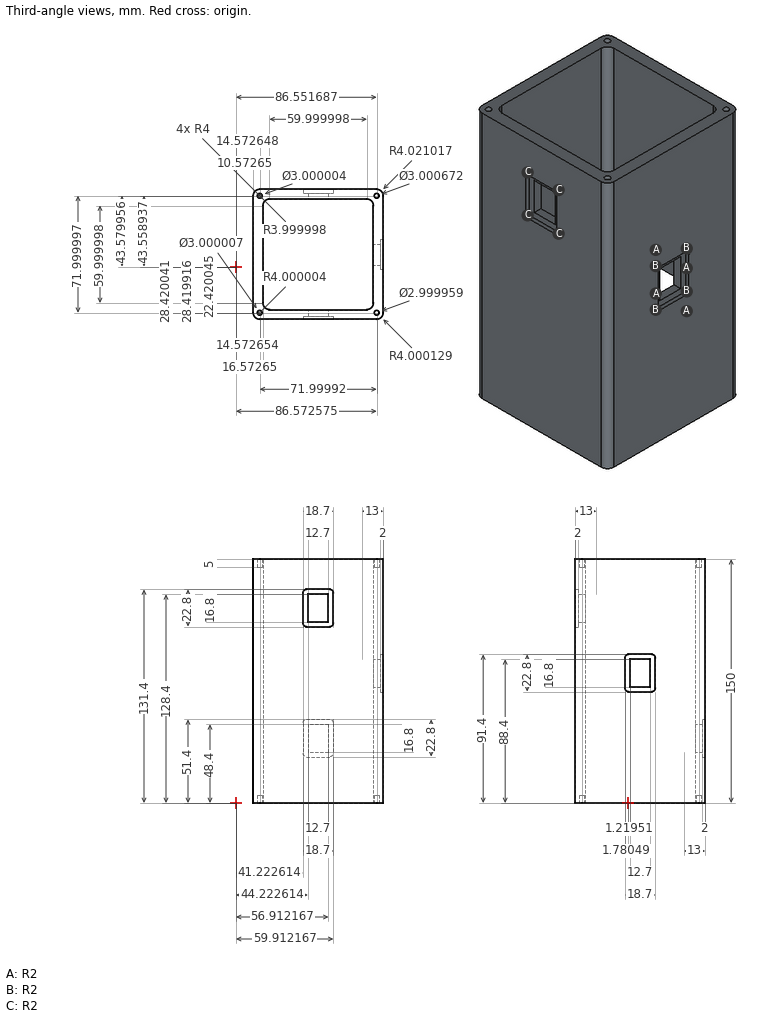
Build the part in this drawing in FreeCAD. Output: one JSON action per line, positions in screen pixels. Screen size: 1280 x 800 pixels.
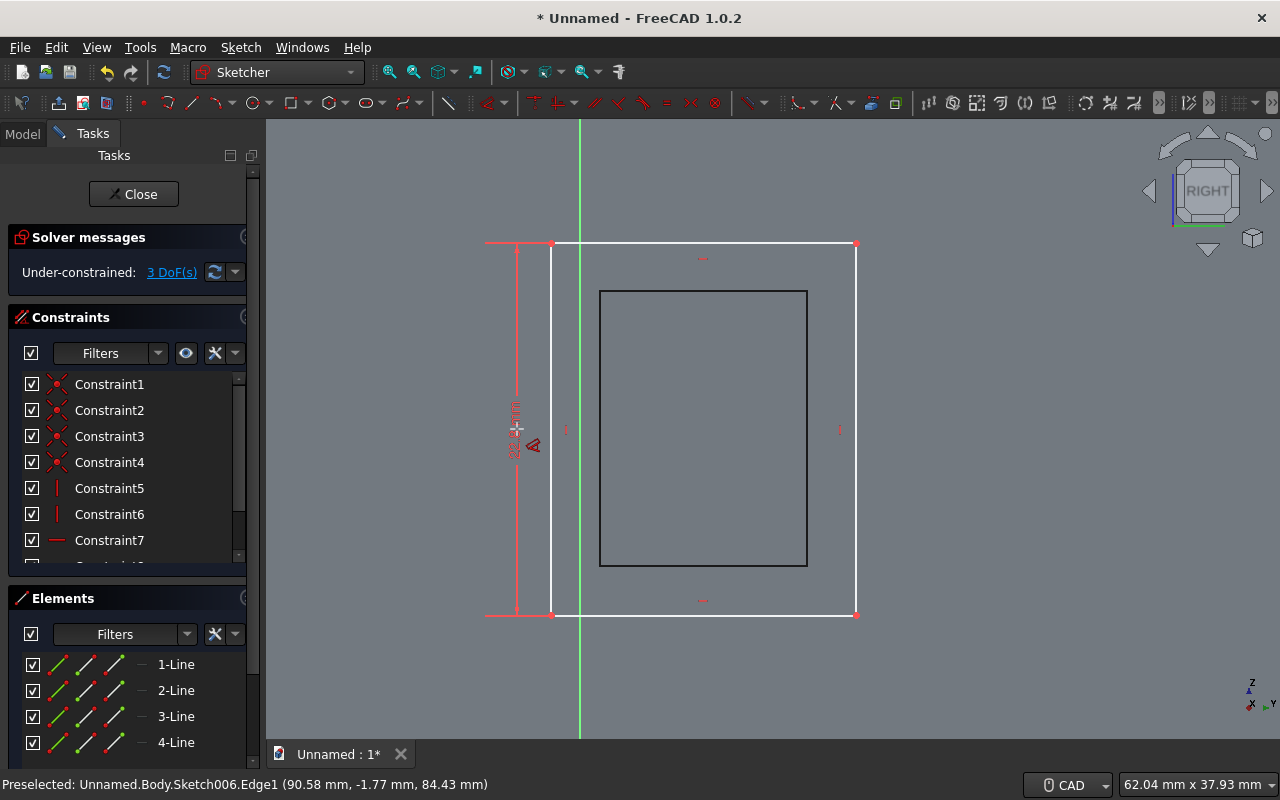
{"action": "left_click", "coordinate": [642, 616]}
{"action": "left_click", "coordinate": [703, 650]}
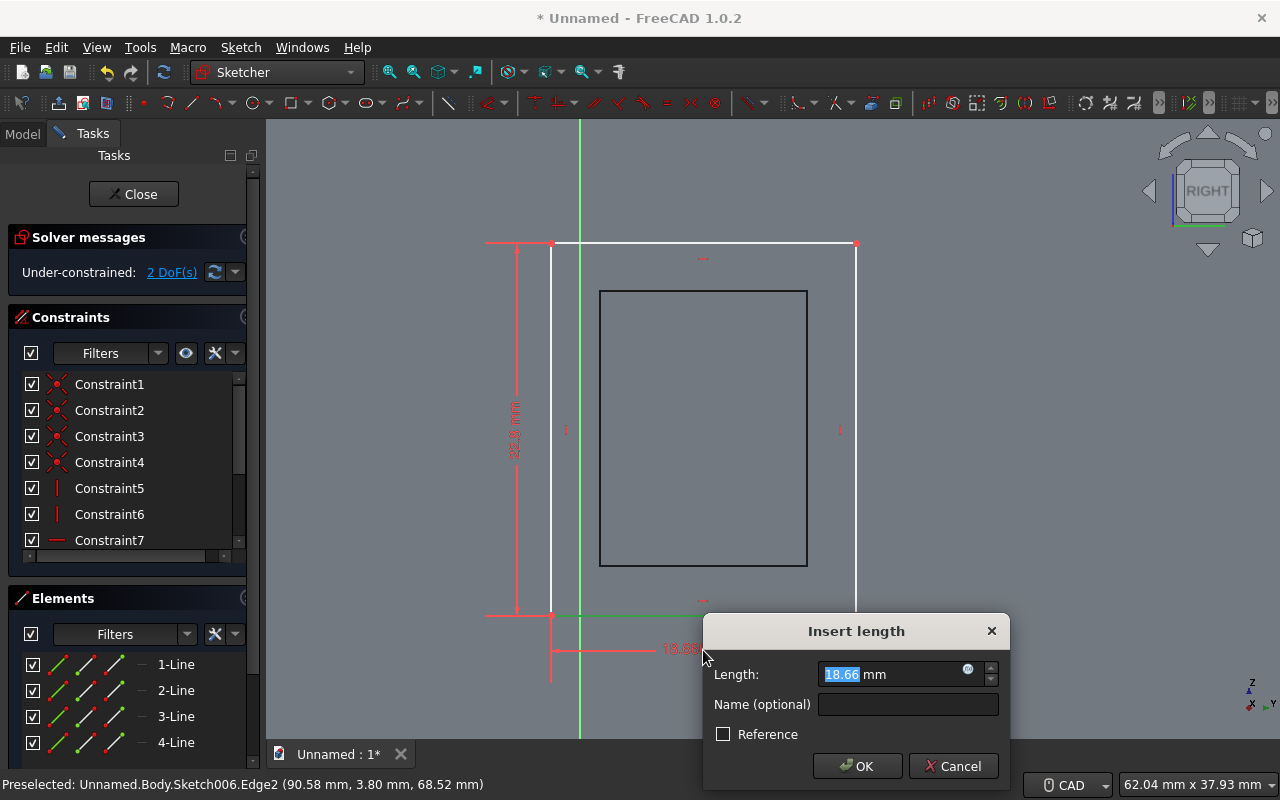
{"action": "type", "text": "18.7"}
{"action": "key", "text": "Return"}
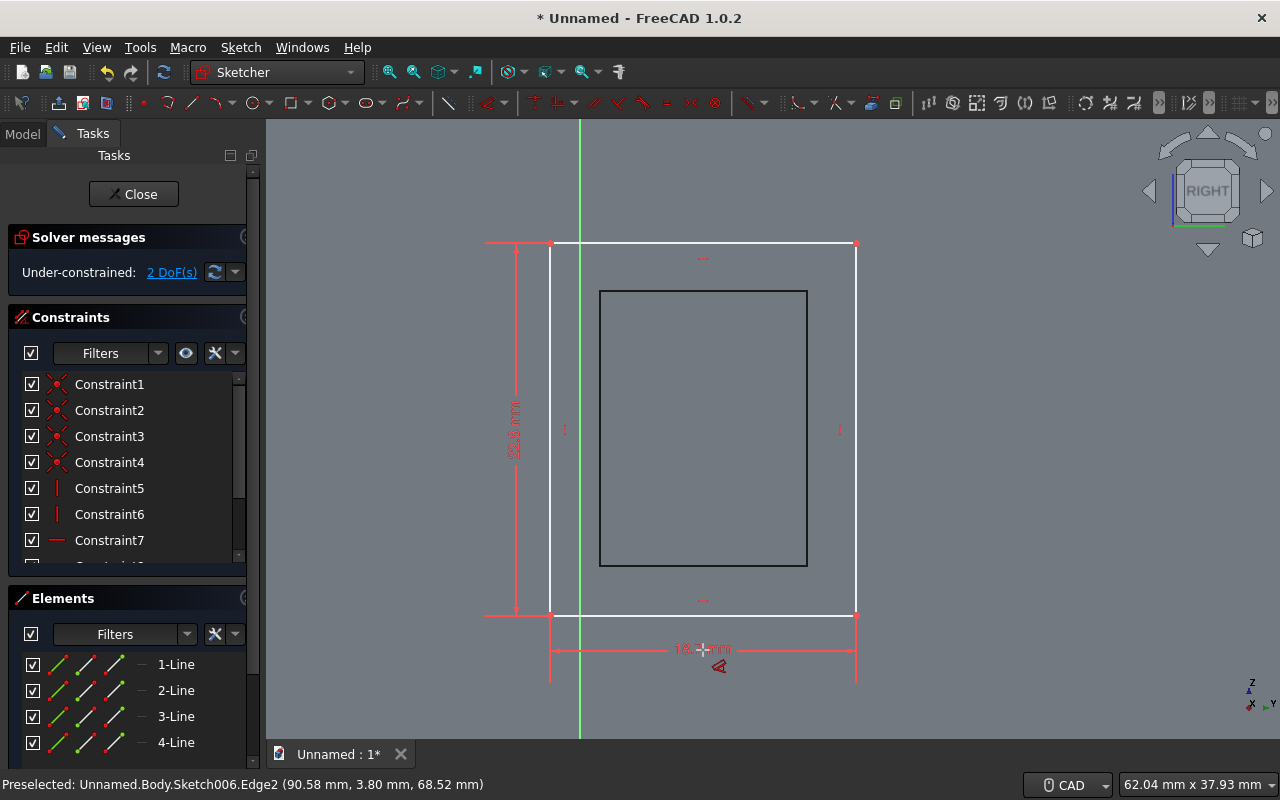
{"action": "left_click", "coordinate": [550, 243]}
{"action": "left_click", "coordinate": [516, 477]}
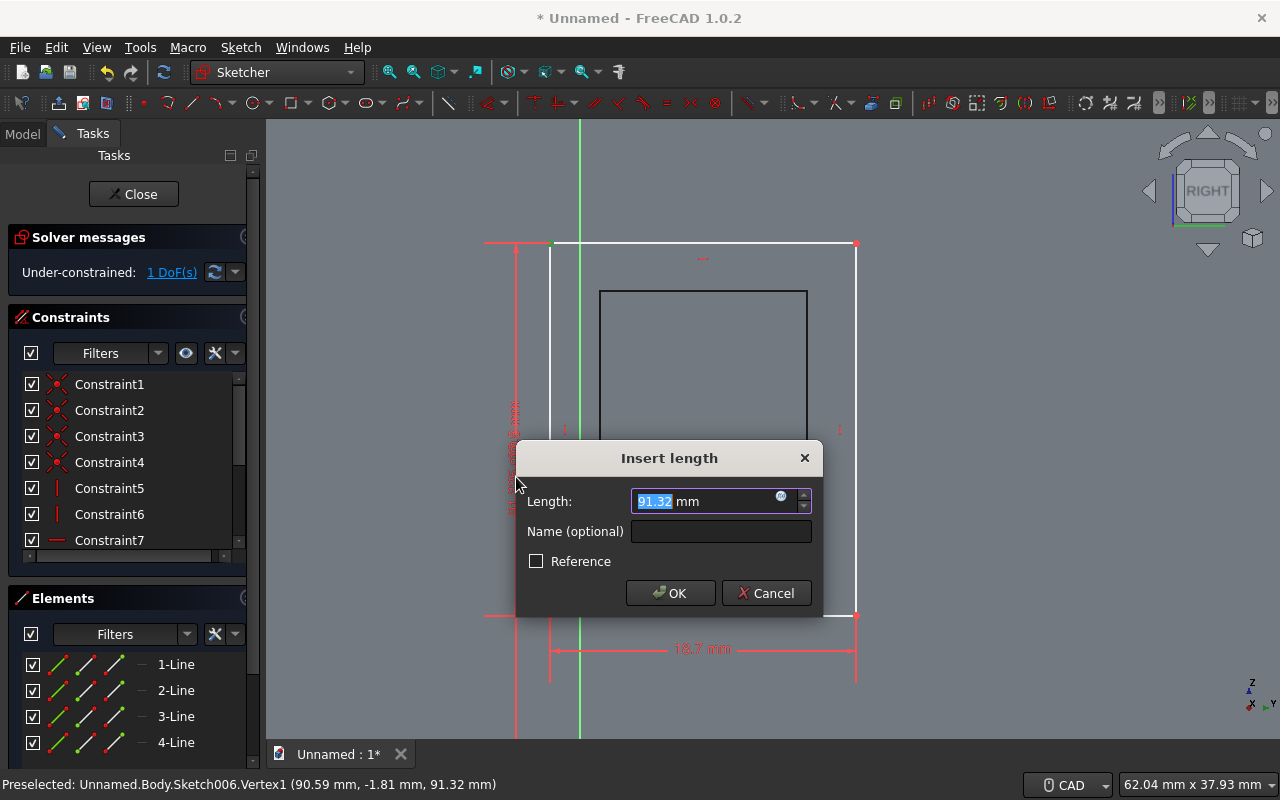
{"action": "type", "text": "91.4"}
{"action": "key", "text": "Return"}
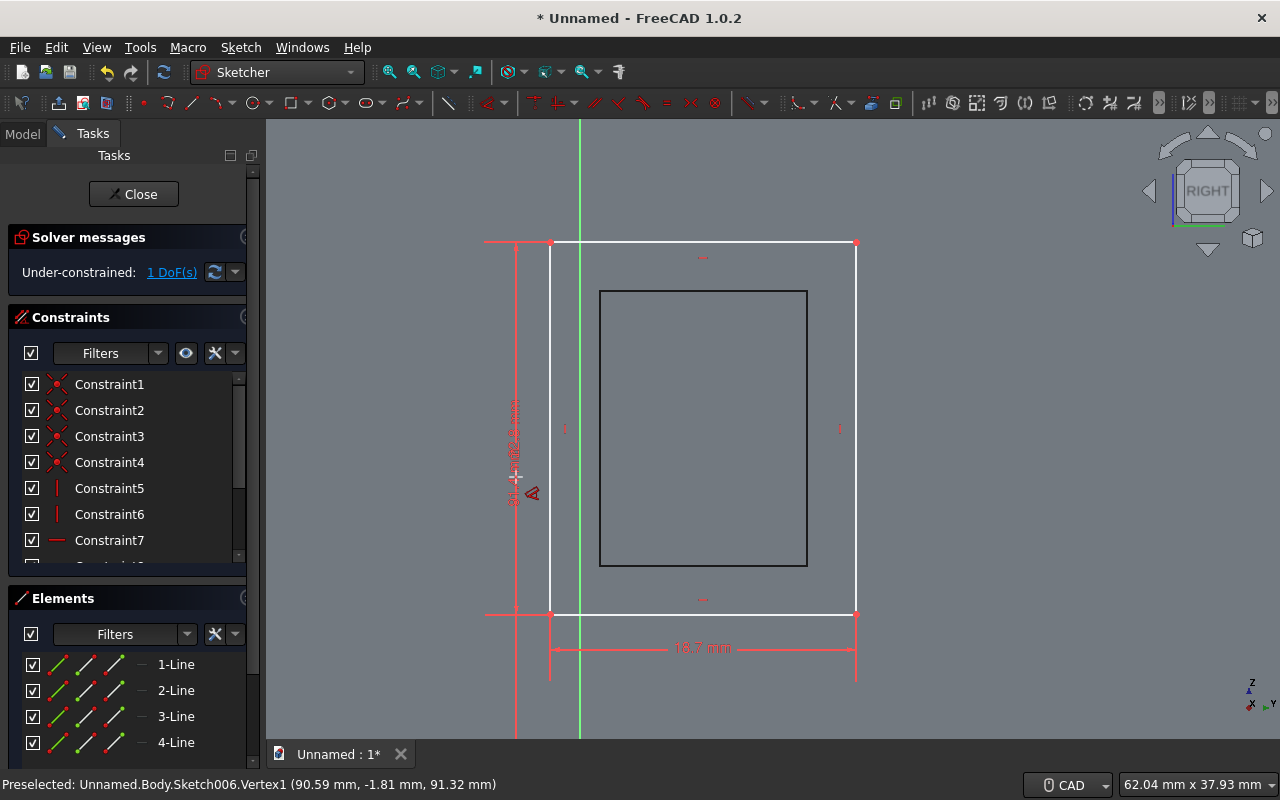
{"action": "scroll", "coordinate": [550, 242], "scroll_direction": "up", "scroll_amount": 2}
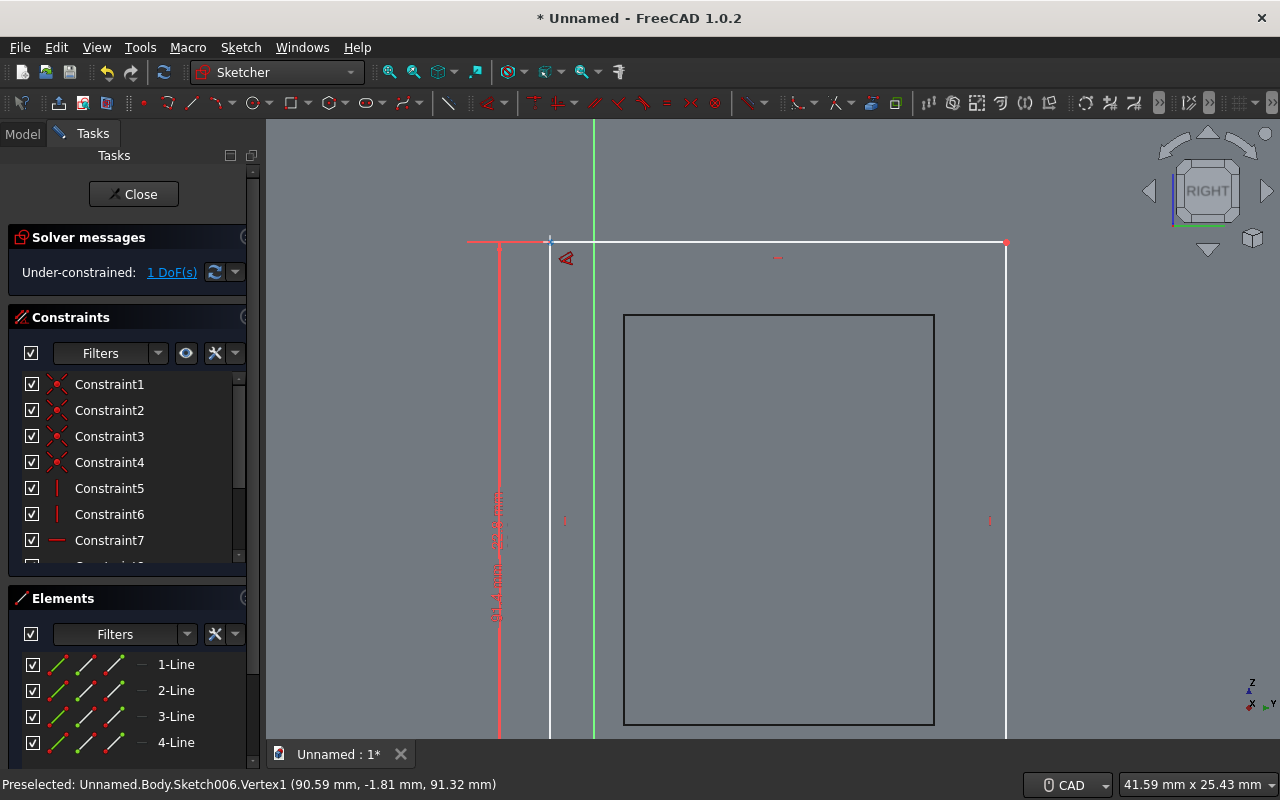
{"action": "left_click", "coordinate": [550, 242]}
{"action": "left_click", "coordinate": [572, 208]}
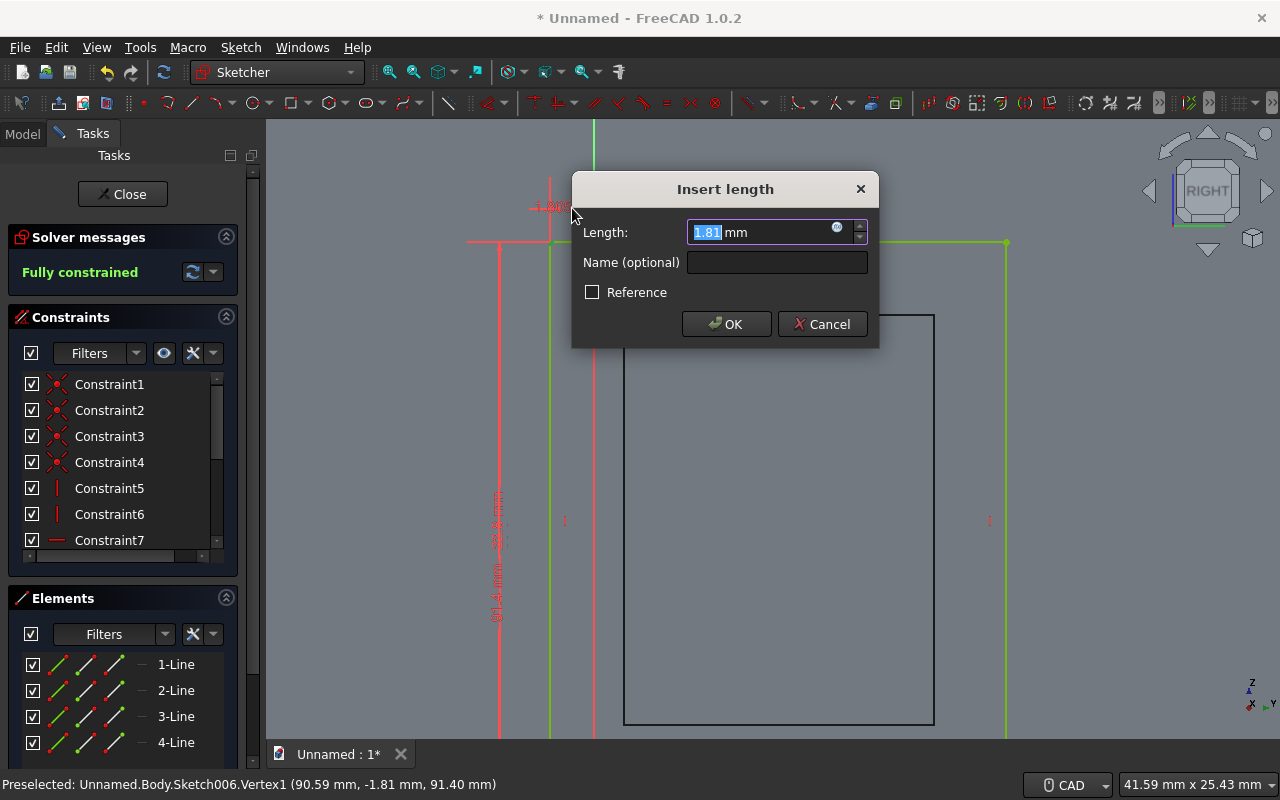
{"action": "type", "text": "1.78049"}
{"action": "key", "text": "Return"}
{"action": "key", "text": "Escape"}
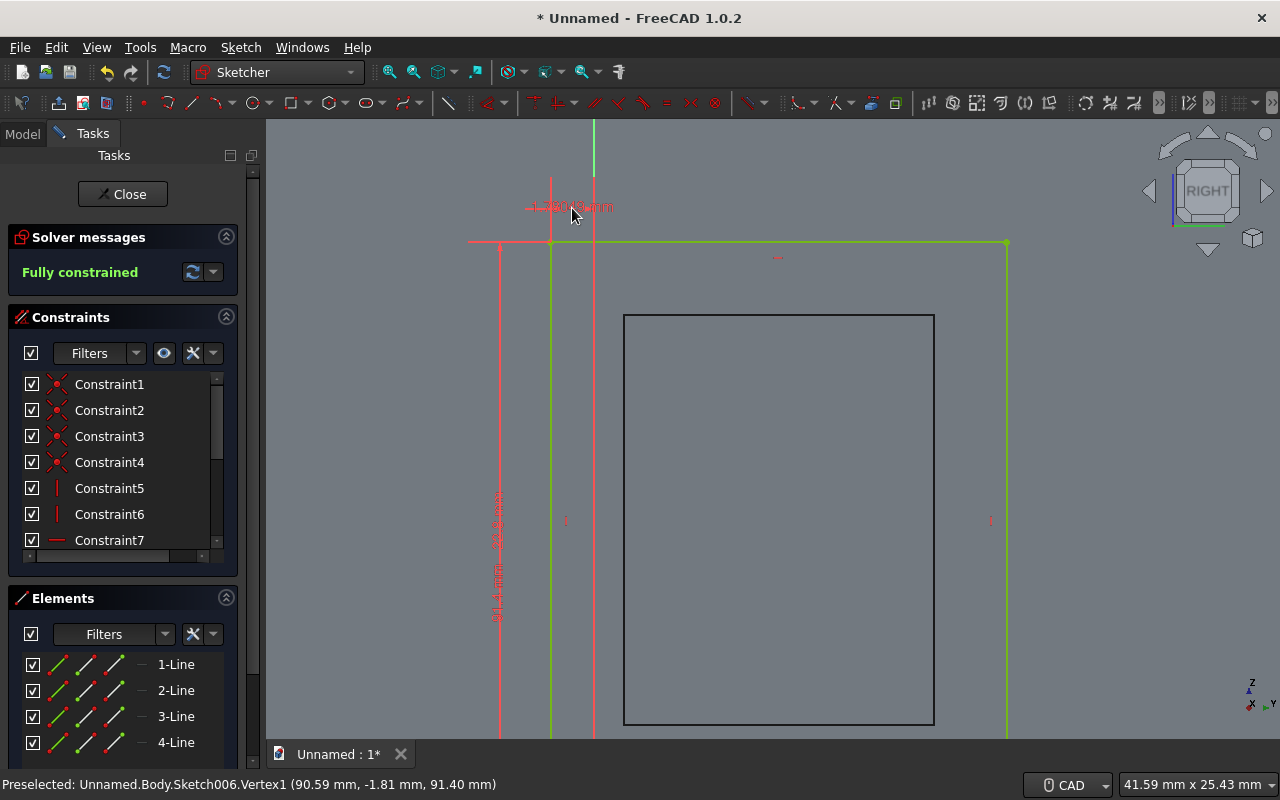
{"action": "left_click", "coordinate": [123, 194]}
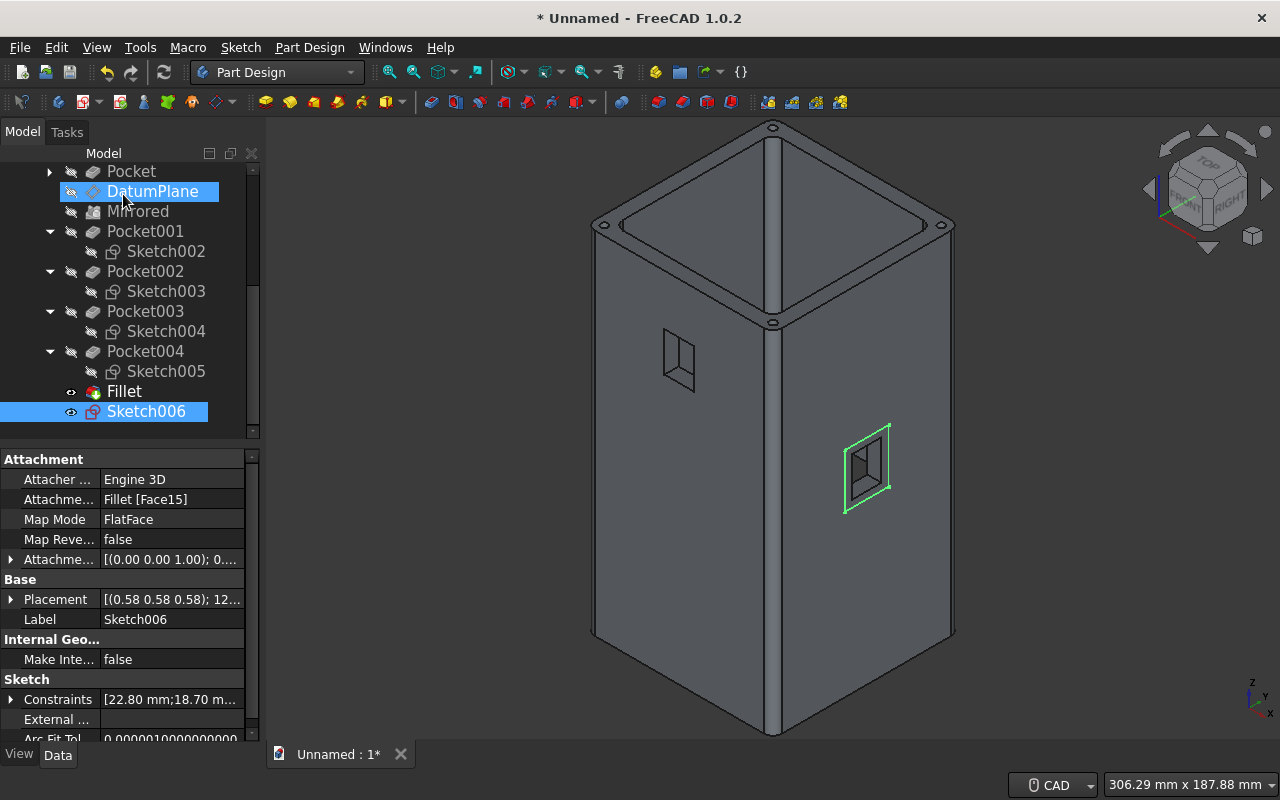
{"action": "left_click", "coordinate": [432, 102]}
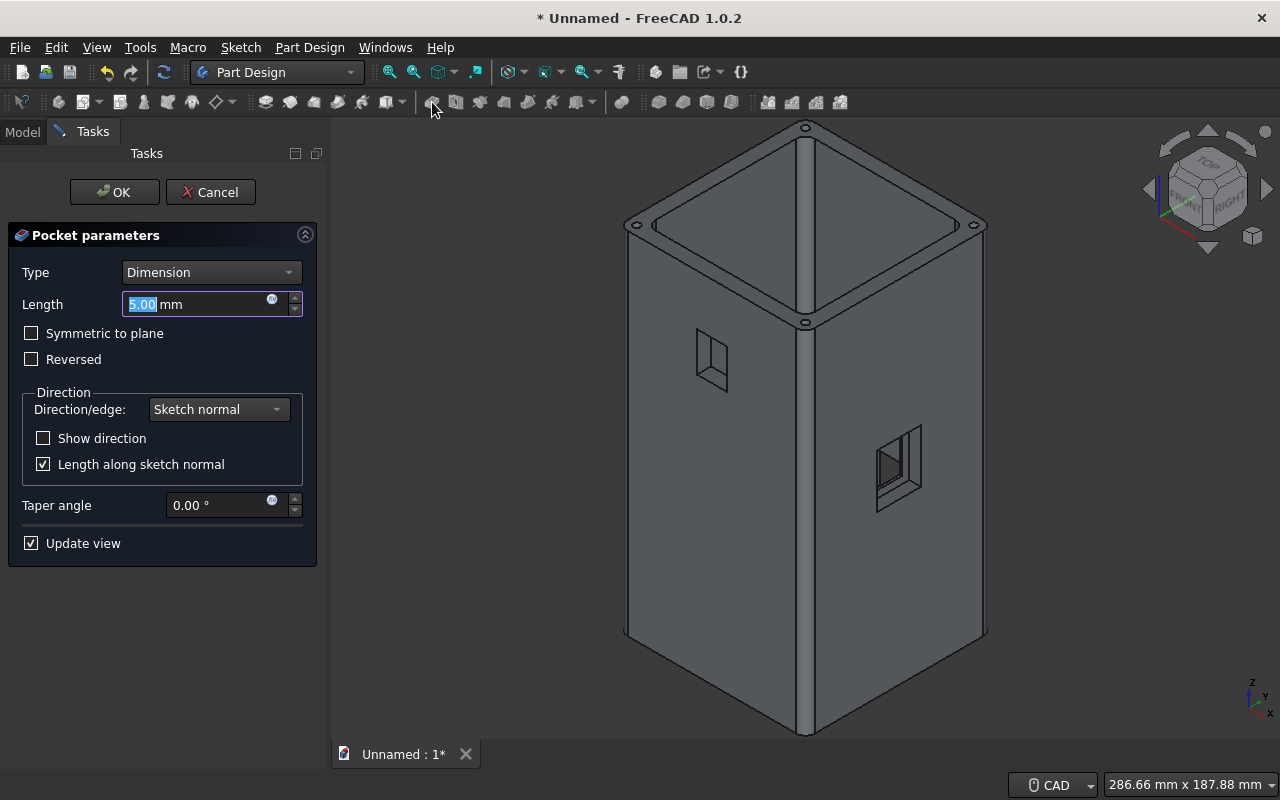
{"action": "type", "text": "2"}
{"action": "key", "text": "Tab"}